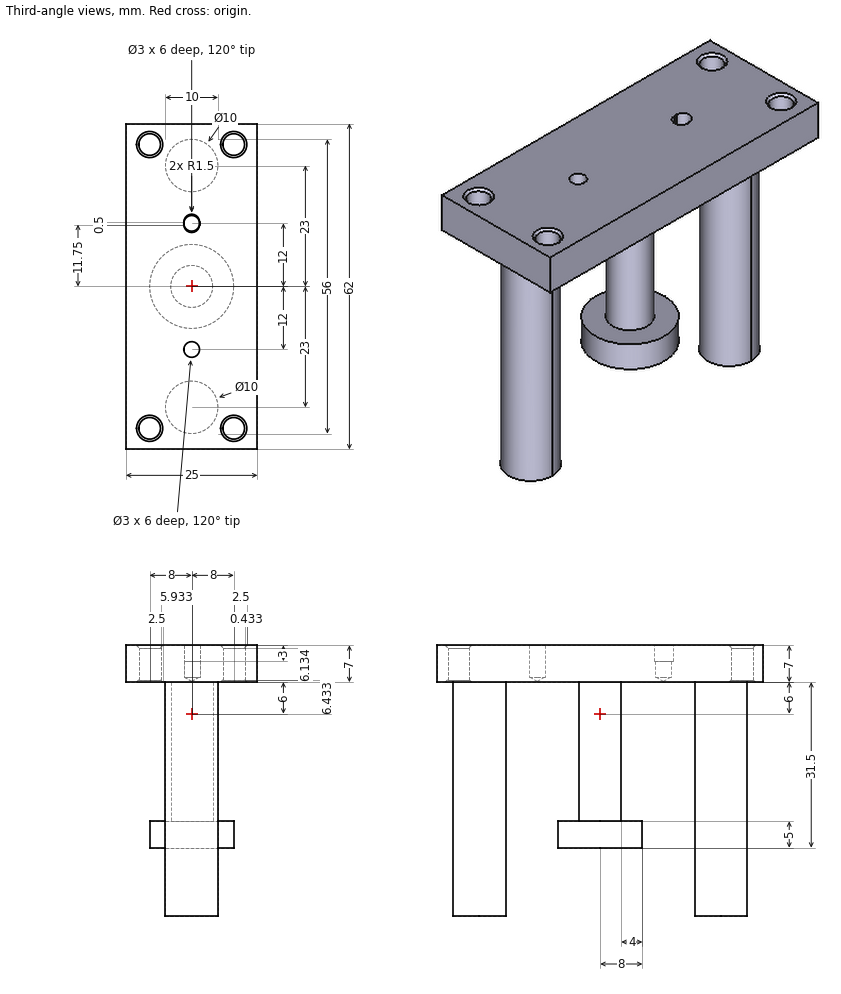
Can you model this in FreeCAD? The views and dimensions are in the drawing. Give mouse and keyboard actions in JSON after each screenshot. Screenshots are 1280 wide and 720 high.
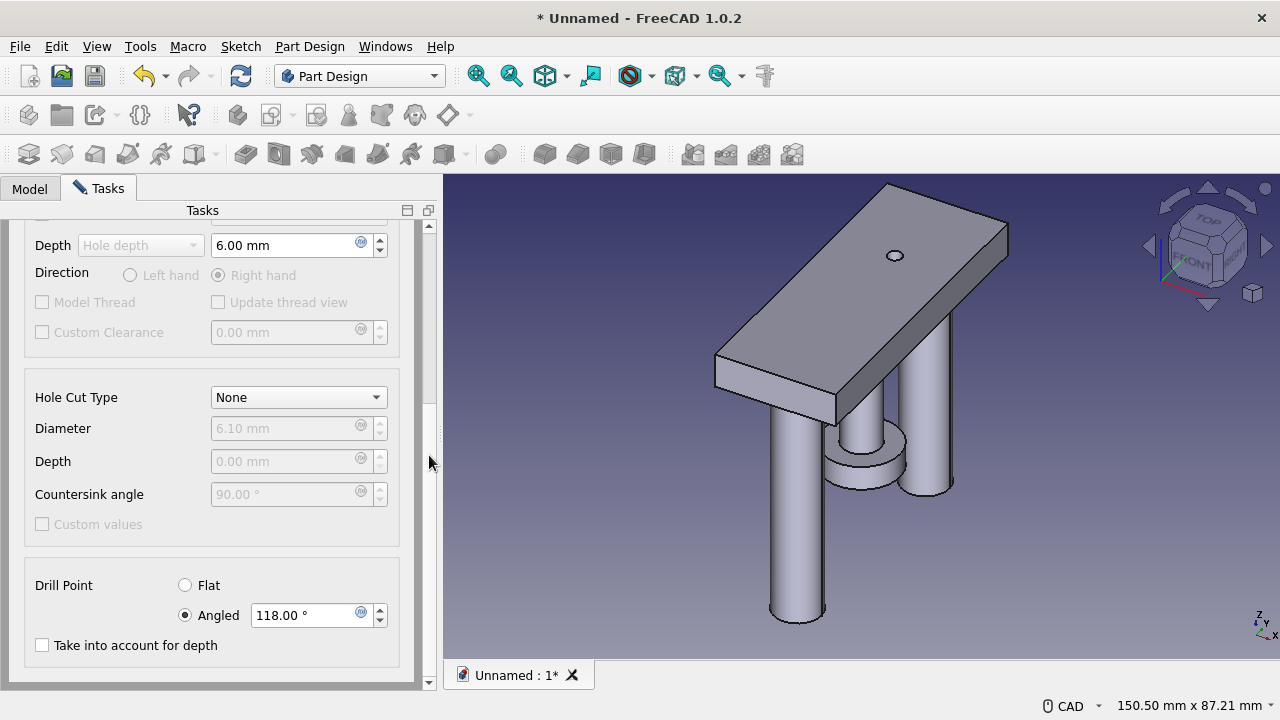
{"action": "triple_click", "coordinate": [312, 616]}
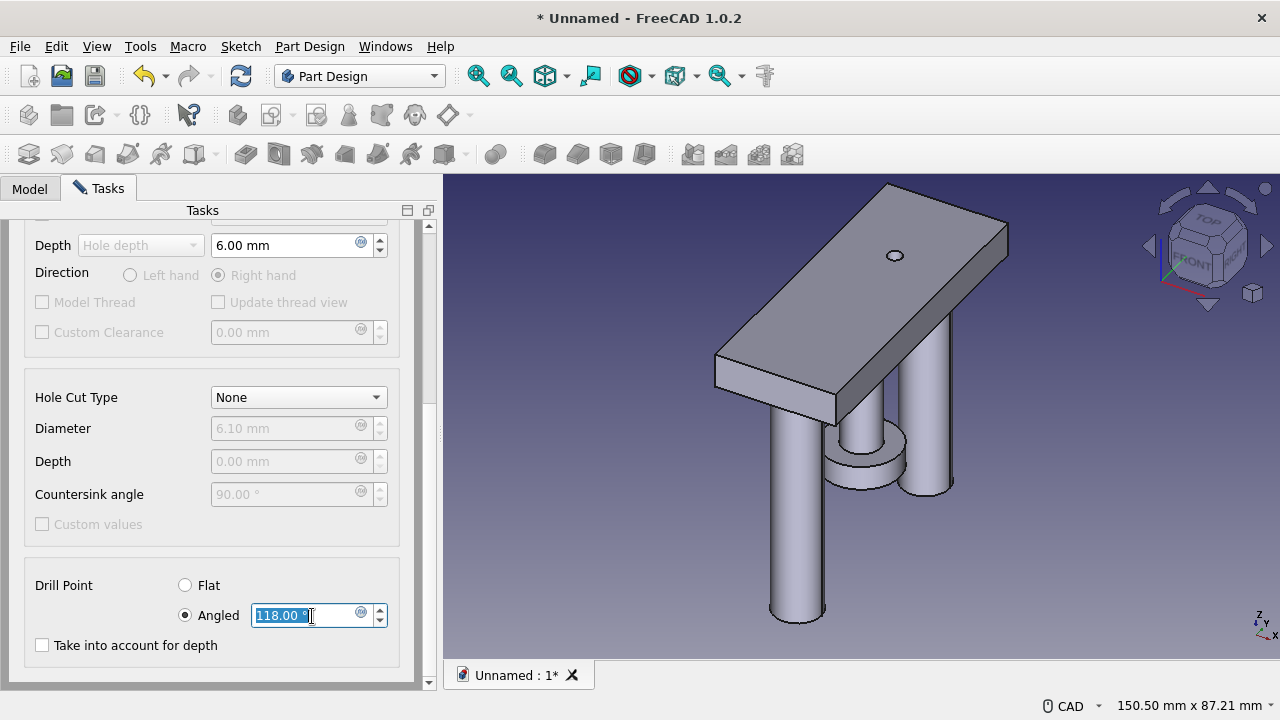
{"action": "type", "text": "120"}
{"action": "key", "text": "Tab"}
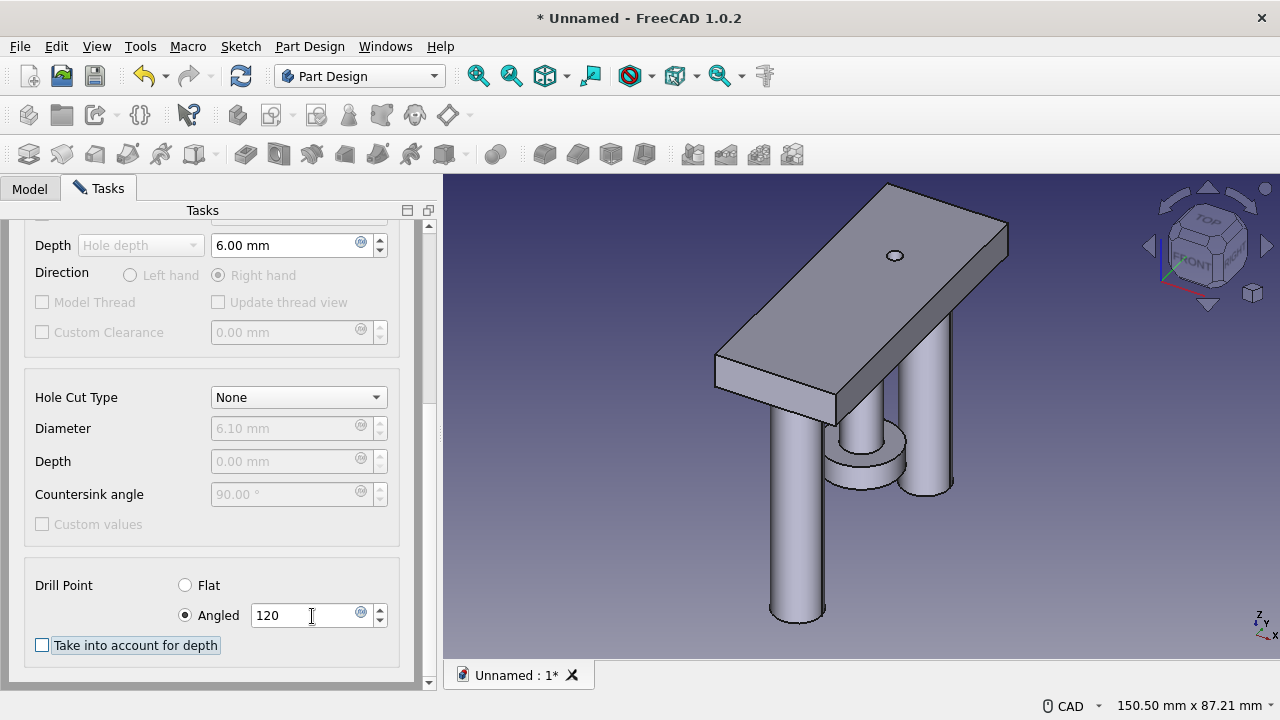
{"action": "scroll", "coordinate": [429, 455], "scroll_direction": "up", "scroll_amount": 6}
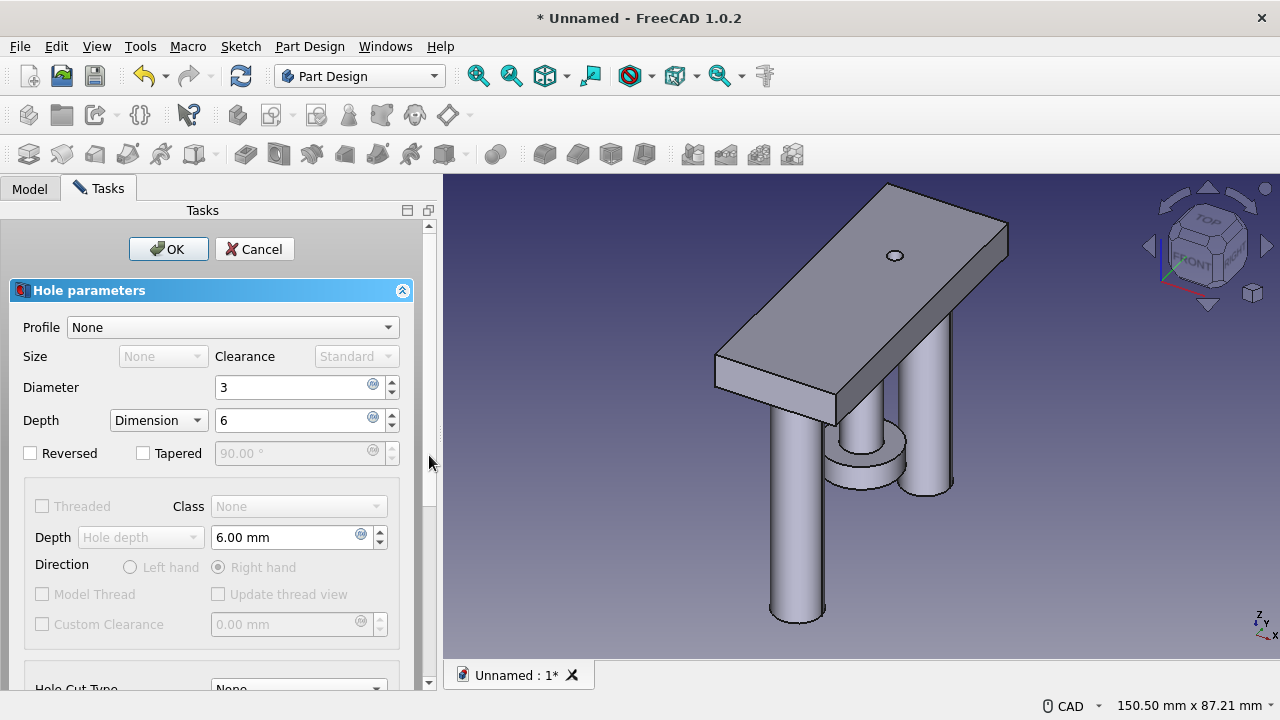
{"action": "left_click", "coordinate": [169, 249]}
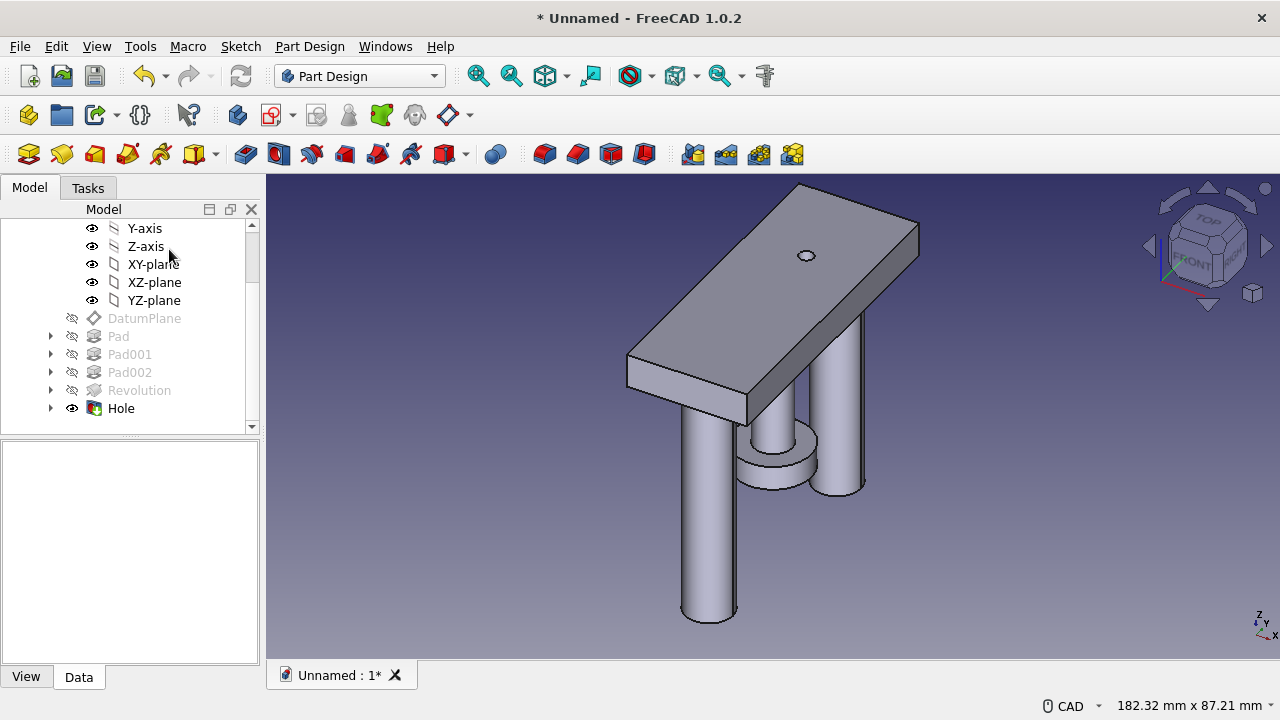
{"action": "left_click", "coordinate": [748, 312]}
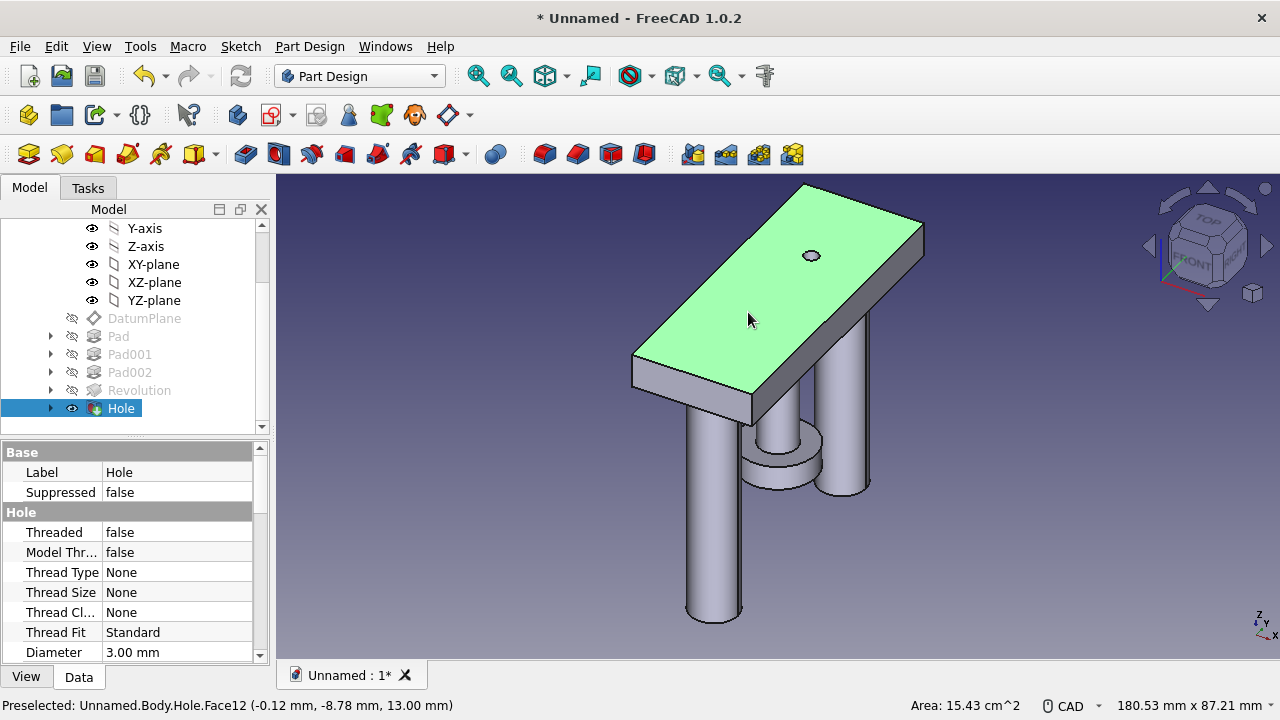
{"action": "left_click", "coordinate": [270, 116]}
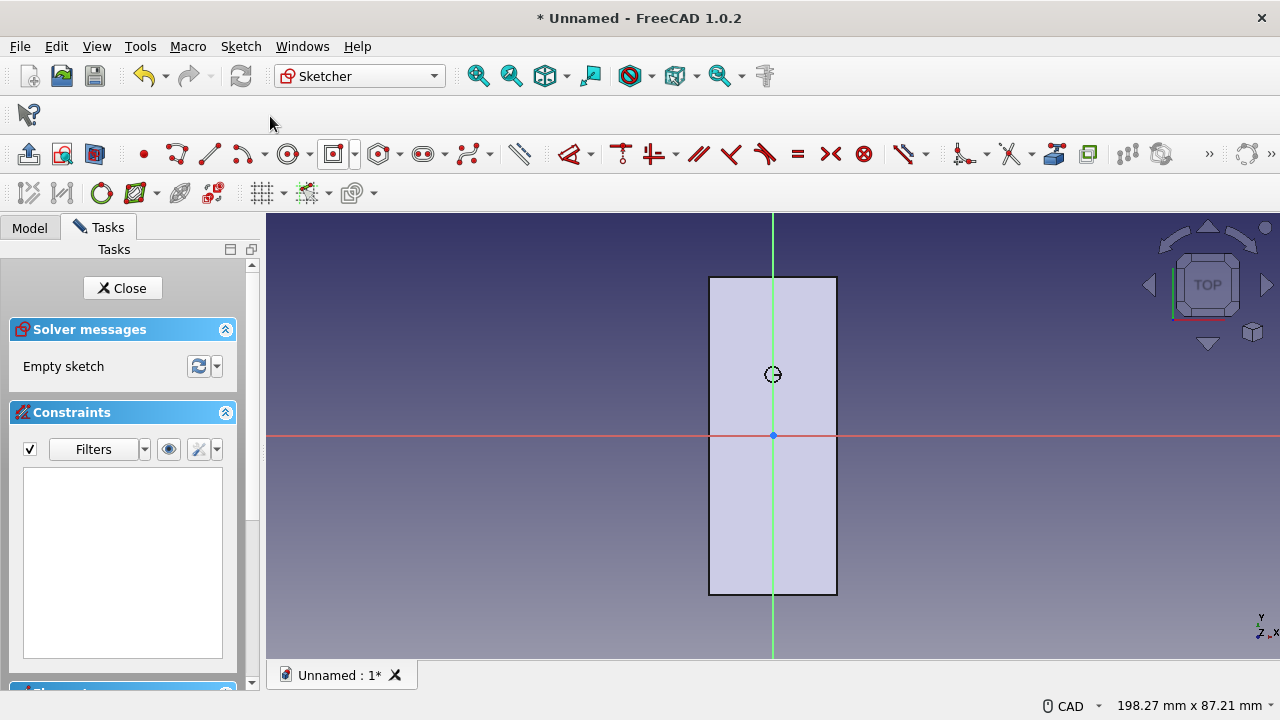
{"action": "scroll", "coordinate": [777, 371], "scroll_direction": "up", "scroll_amount": 14}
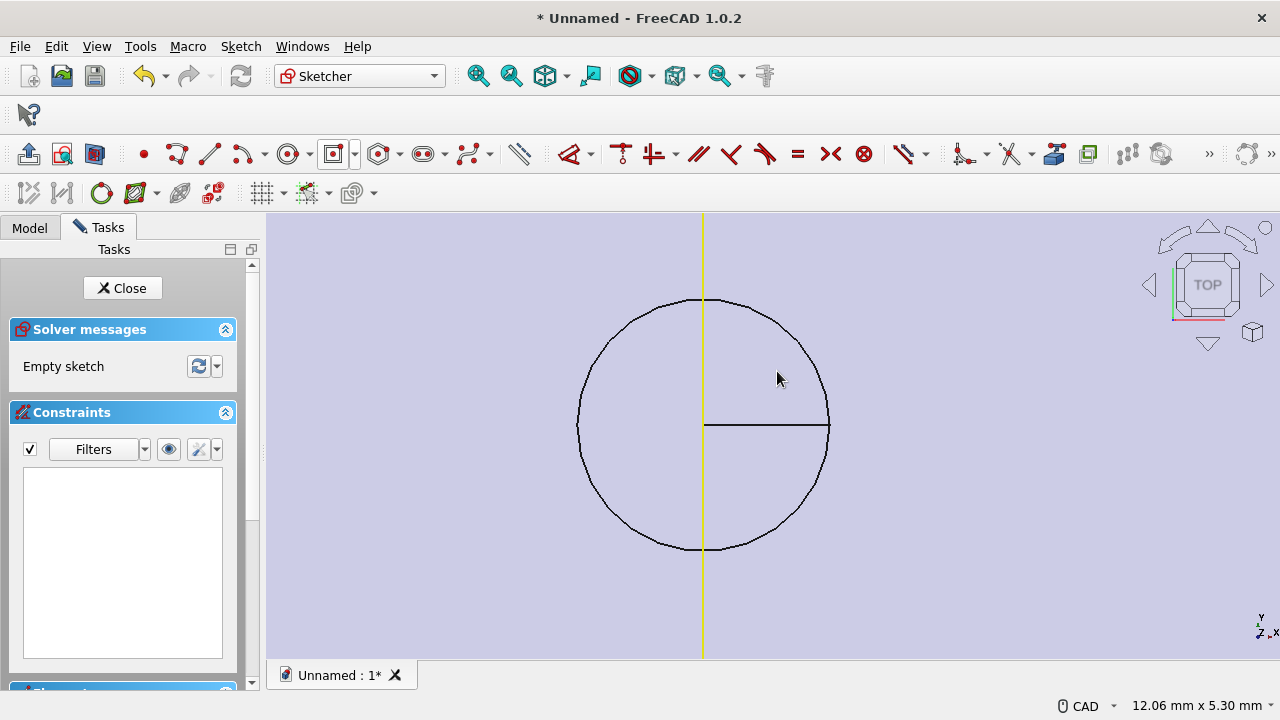
{"action": "left_click", "coordinate": [422, 154]}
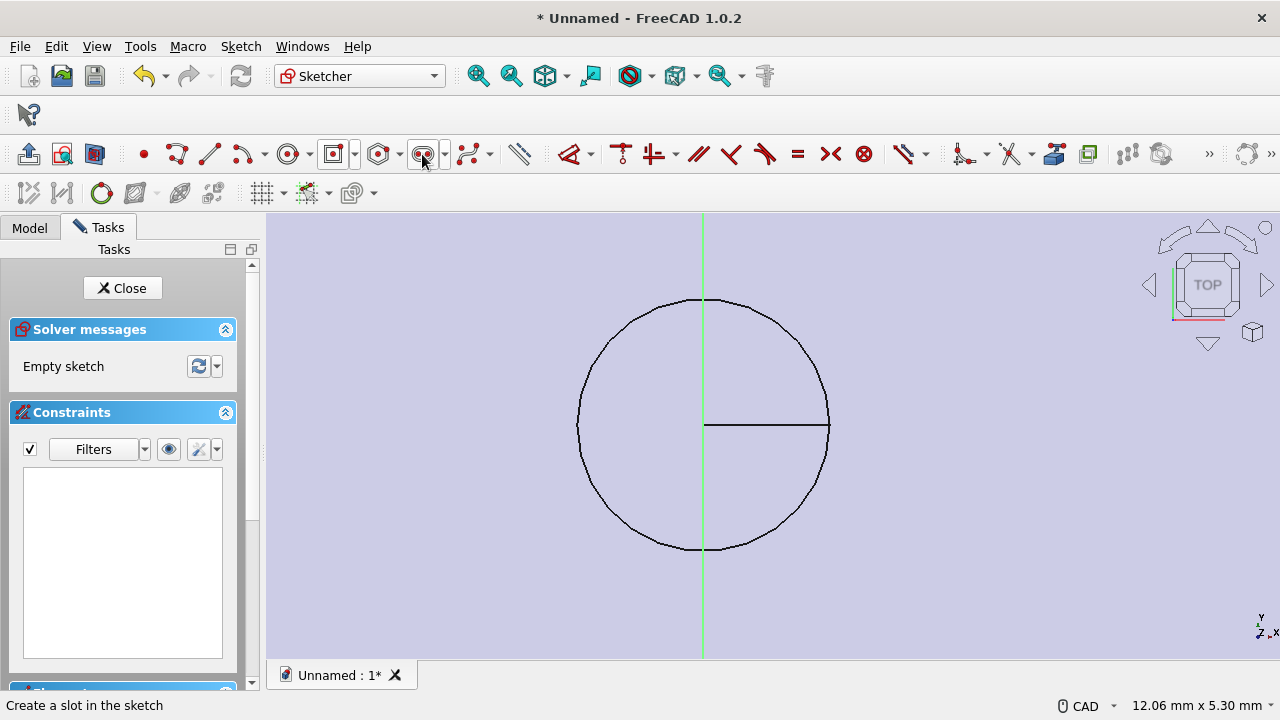
{"action": "left_click", "coordinate": [703, 446]}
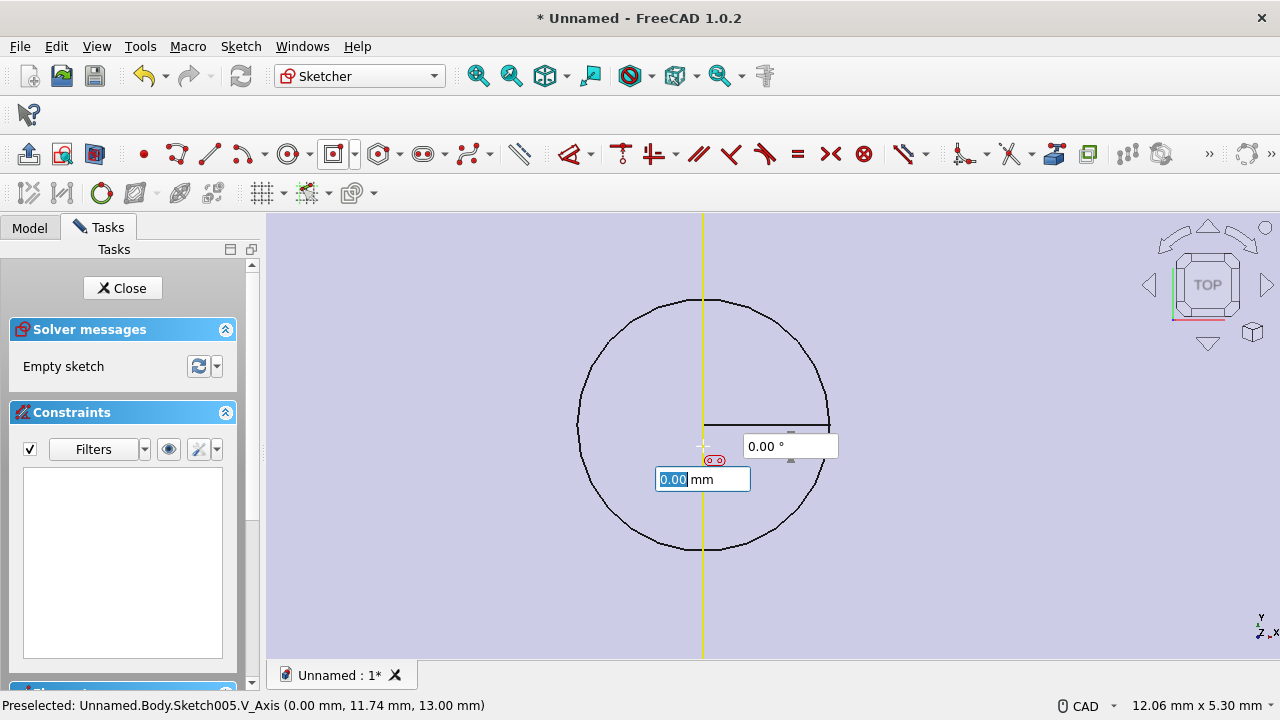
{"action": "left_click", "coordinate": [712, 404]}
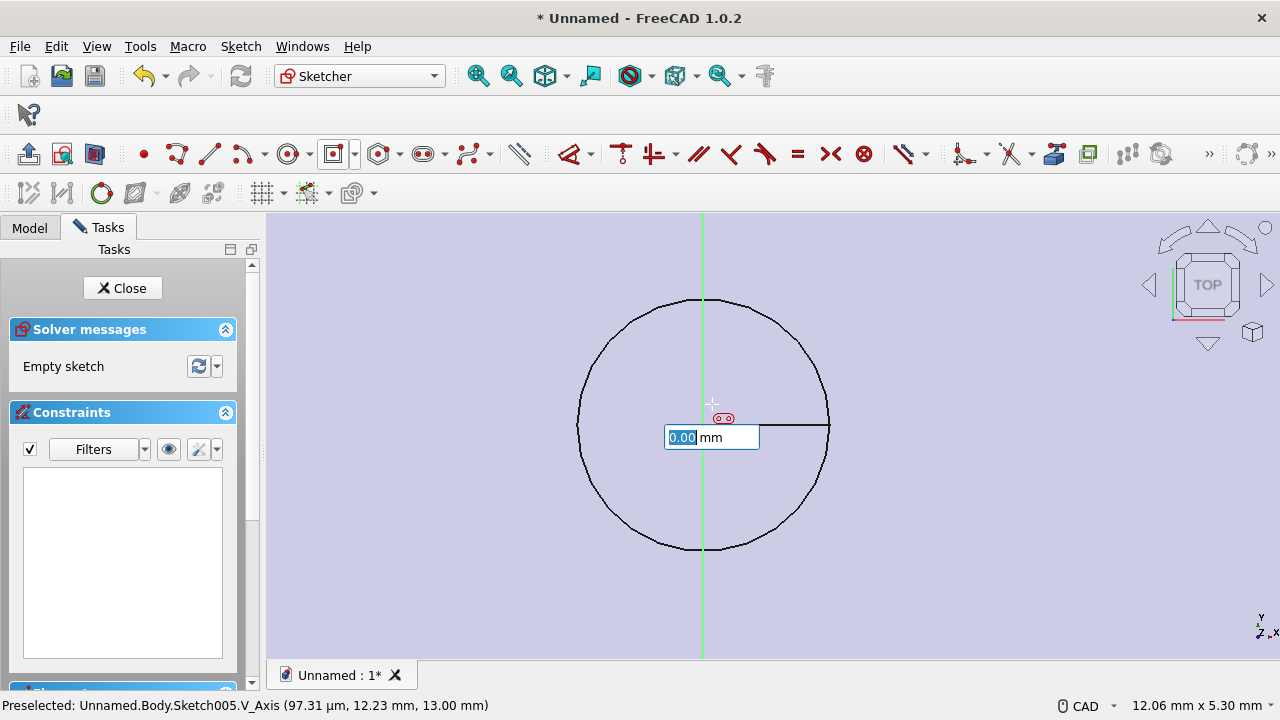
{"action": "left_click", "coordinate": [830, 425]}
{"action": "key", "text": "Escape"}